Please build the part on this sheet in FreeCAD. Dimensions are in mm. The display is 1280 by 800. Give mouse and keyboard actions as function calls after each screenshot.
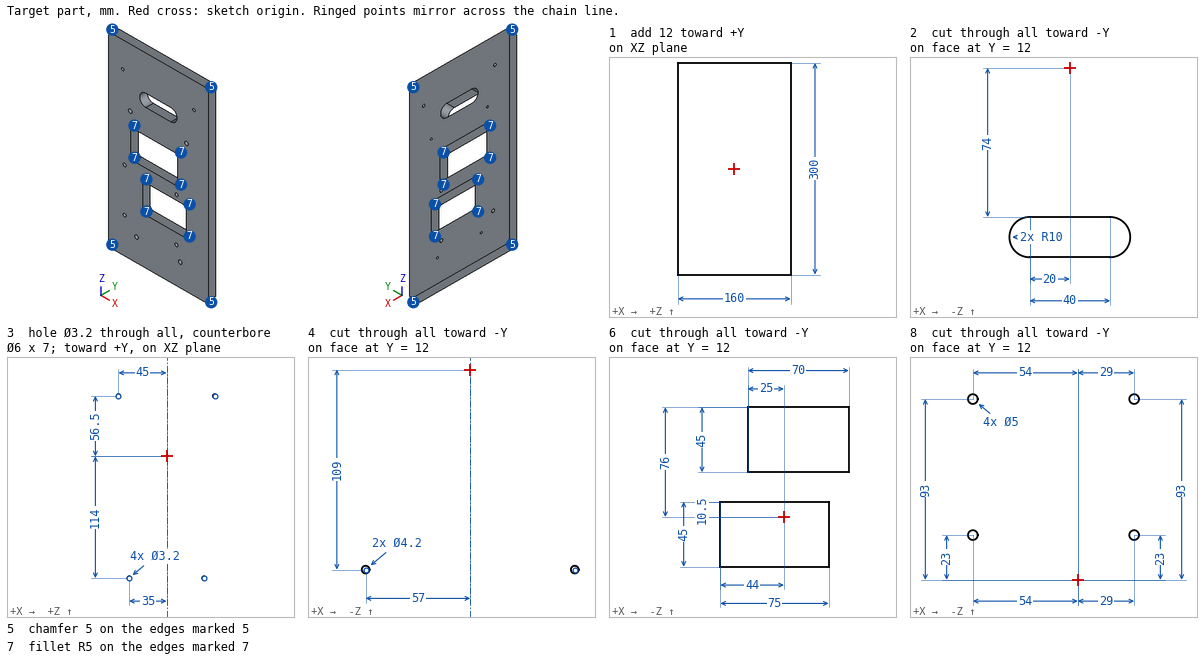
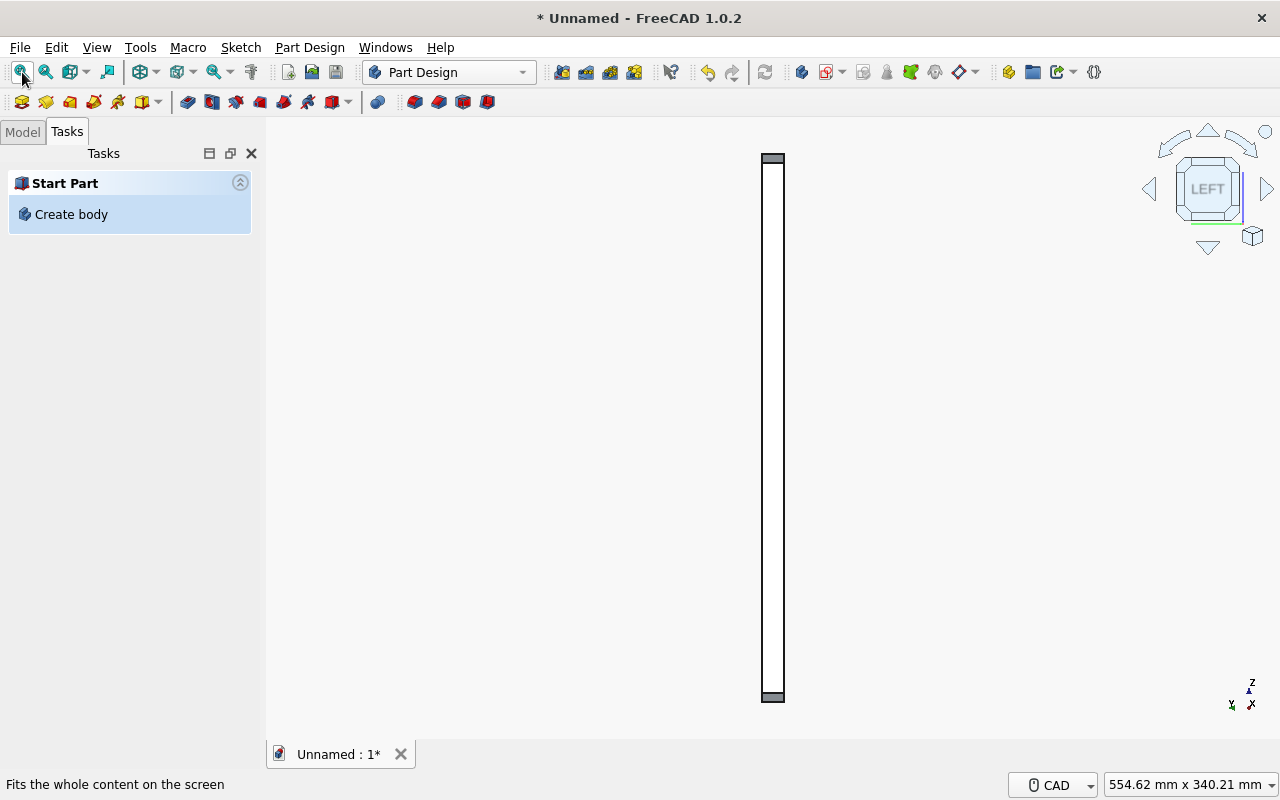
key(0)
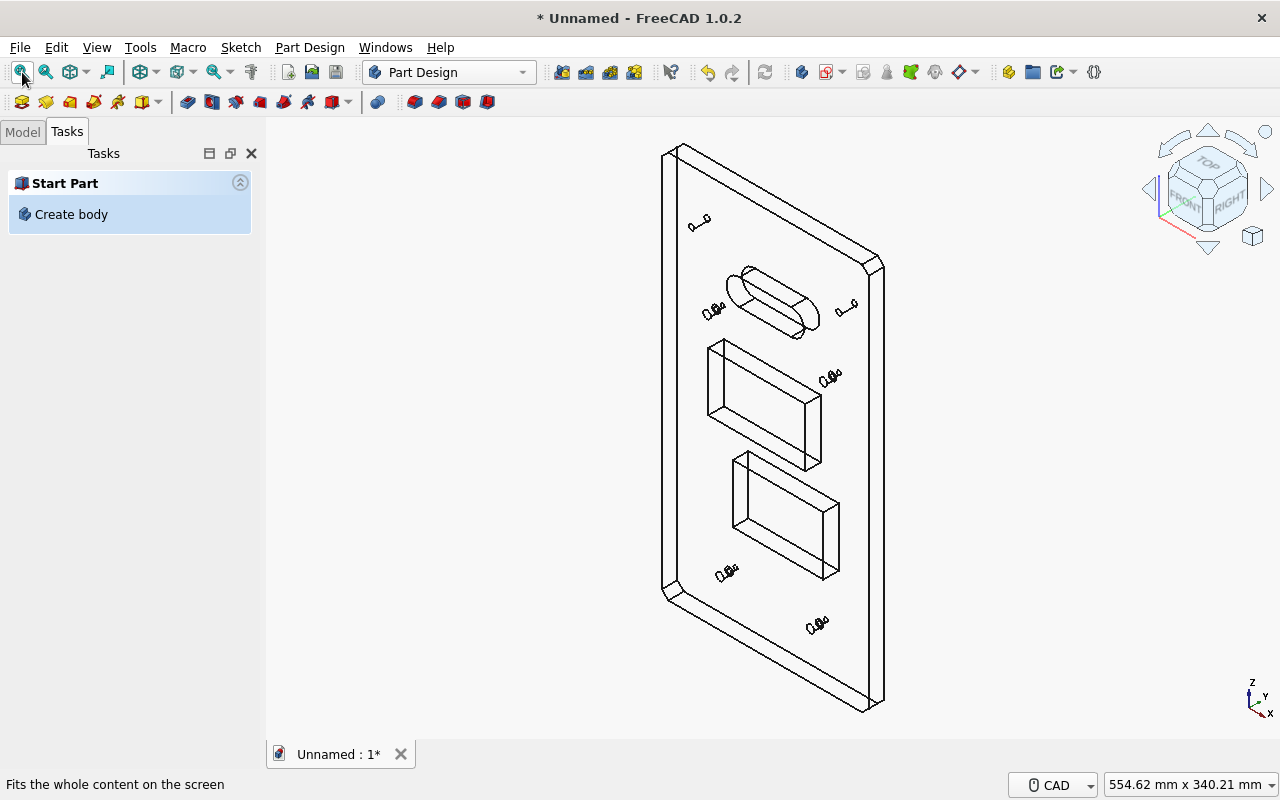
click(813, 466)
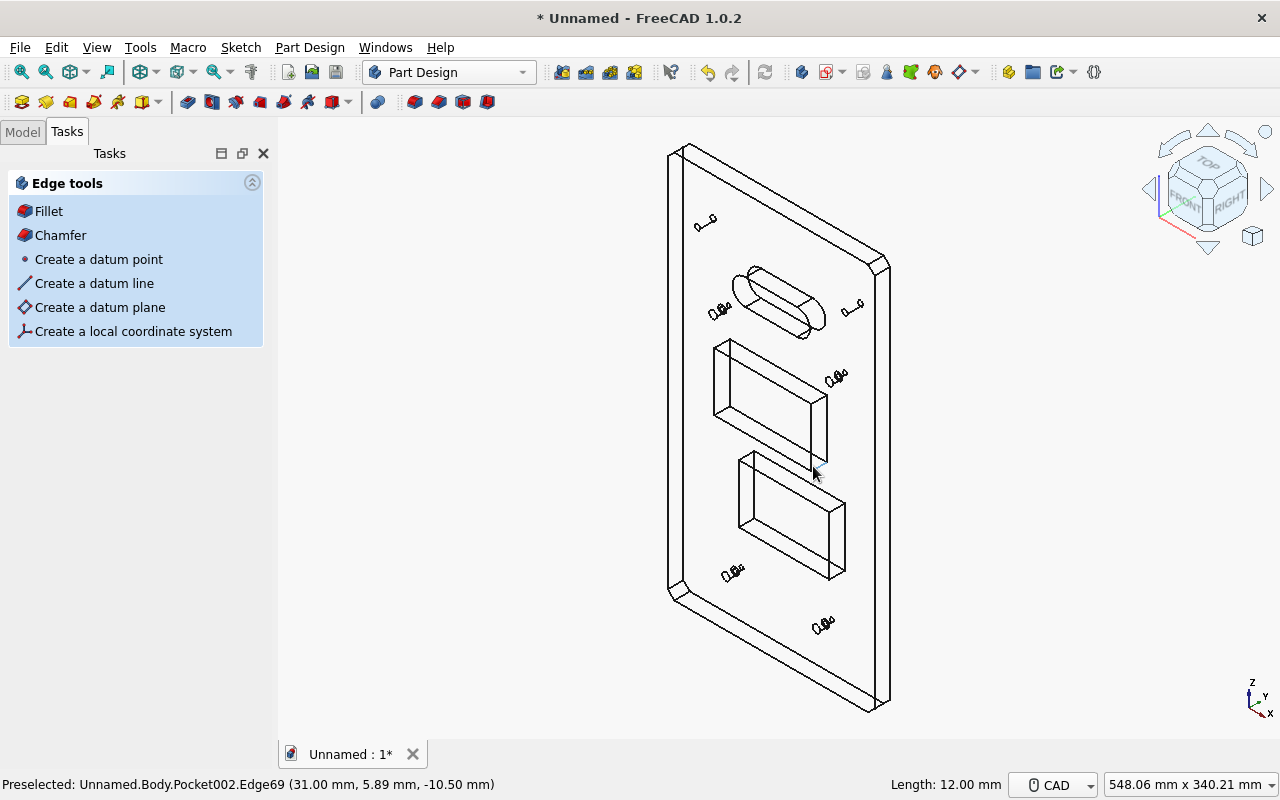
click(819, 399, ctrl)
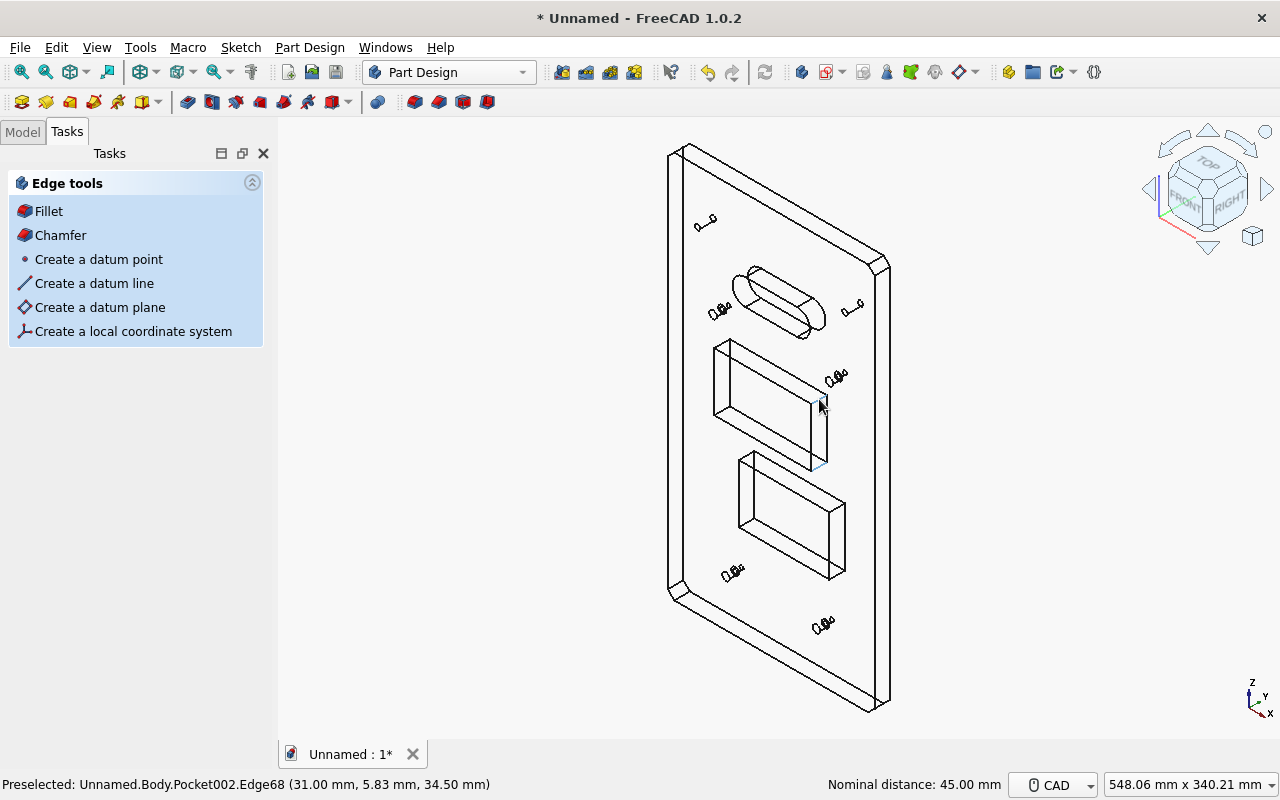
click(722, 343, ctrl)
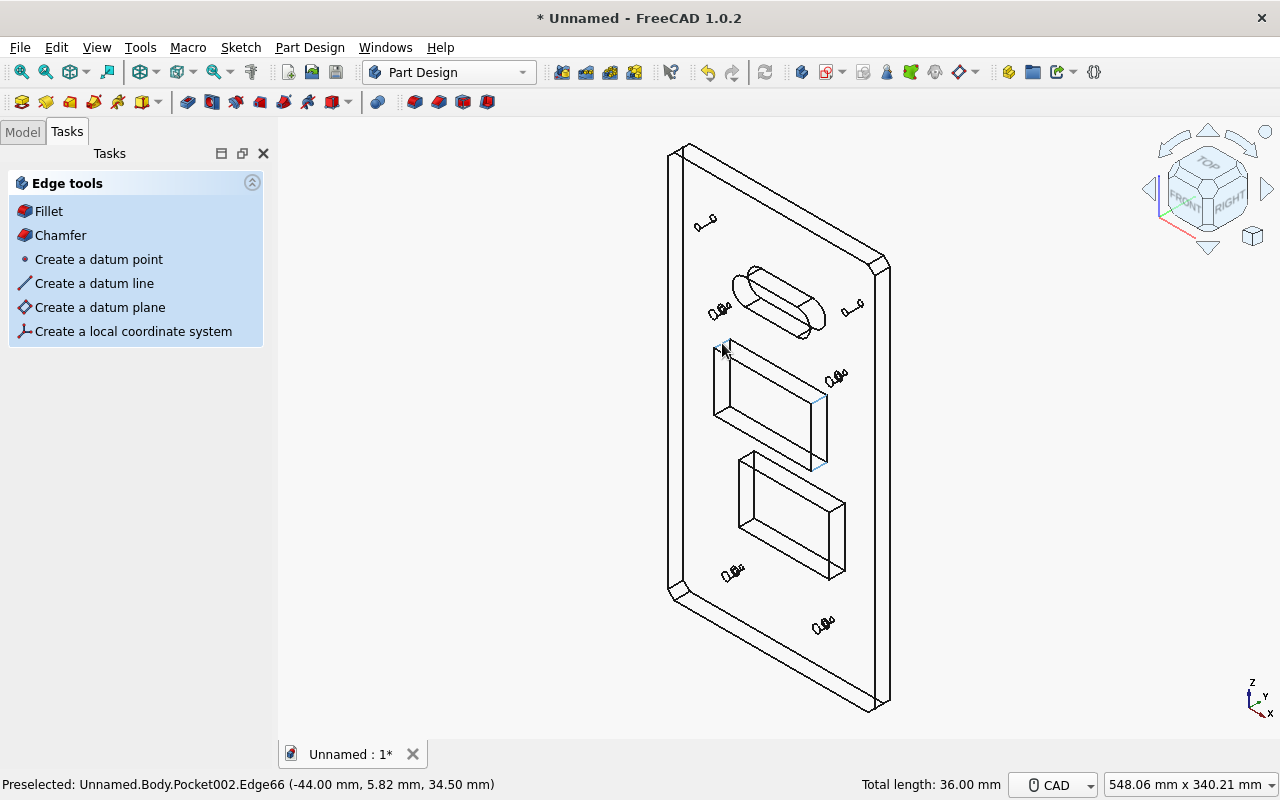
click(722, 410, ctrl)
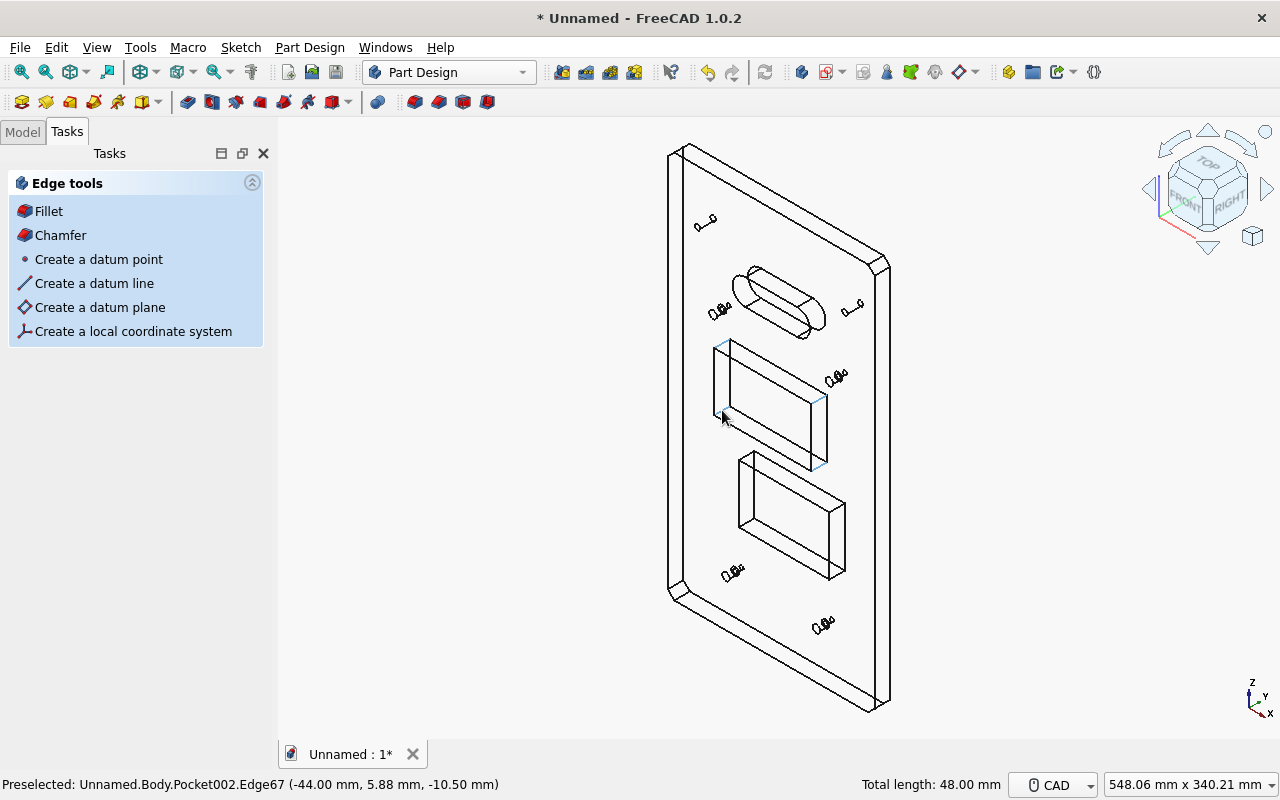
click(837, 574, ctrl)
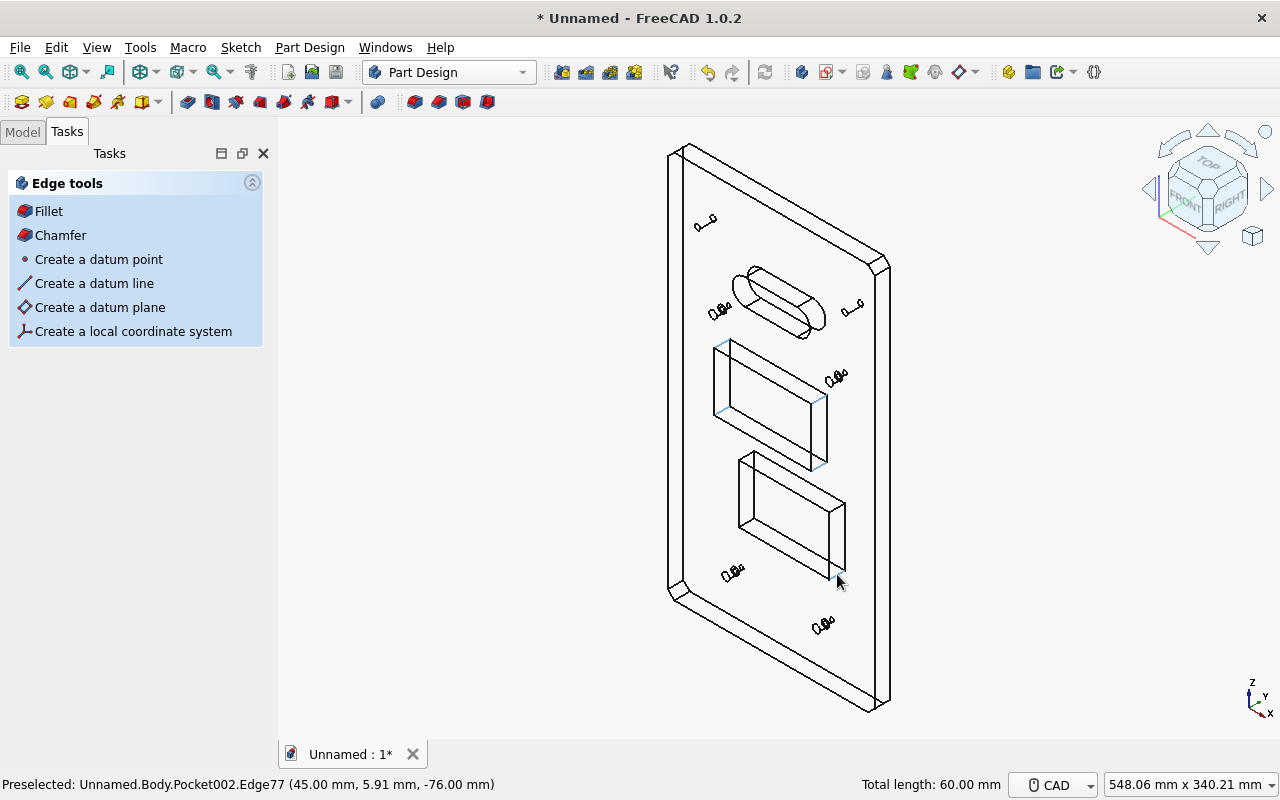
click(837, 507, ctrl)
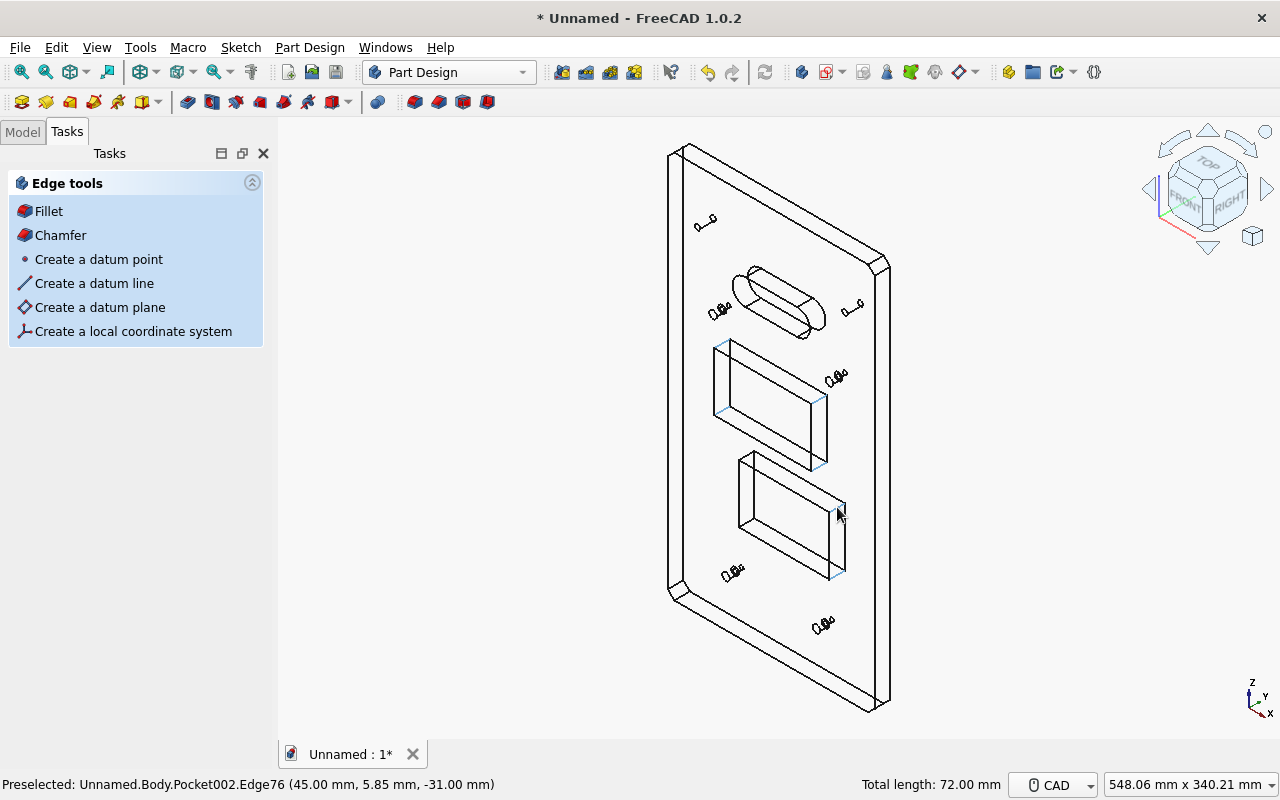
click(747, 455, ctrl)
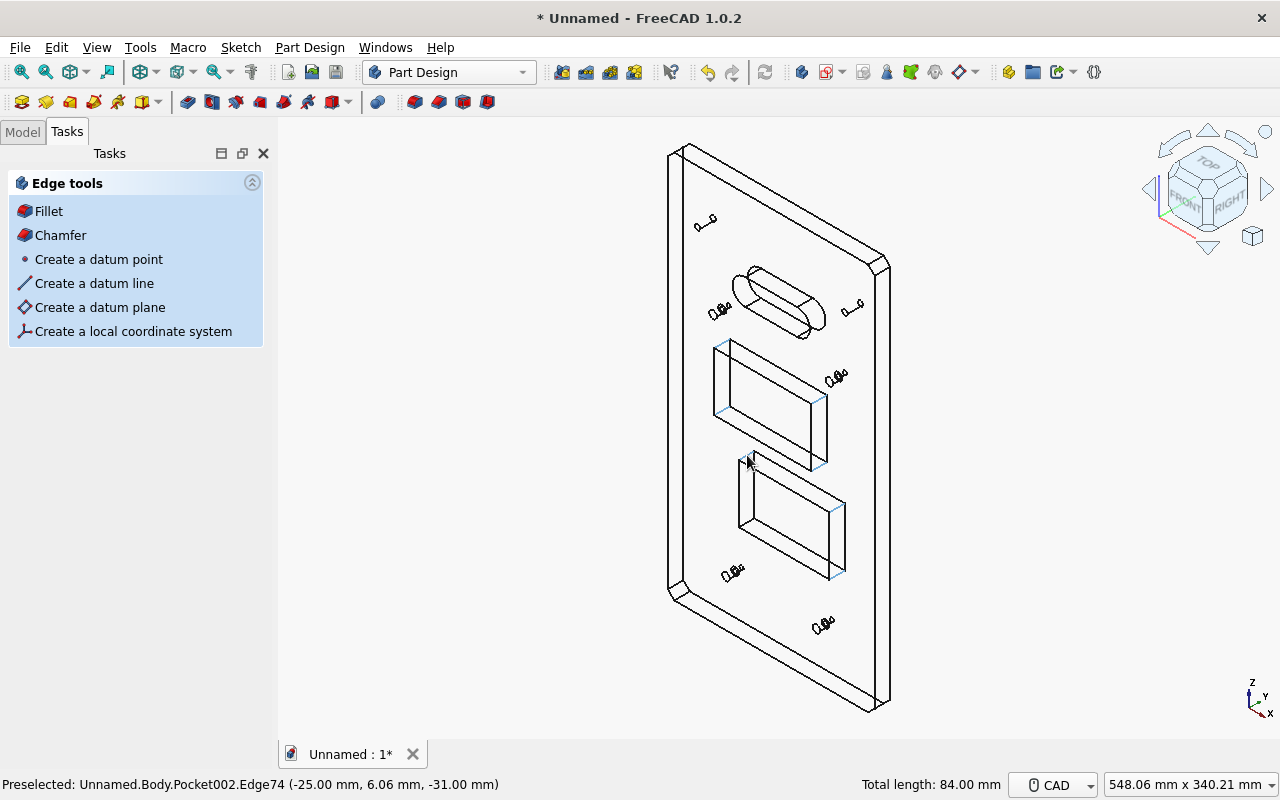
click(747, 522, ctrl)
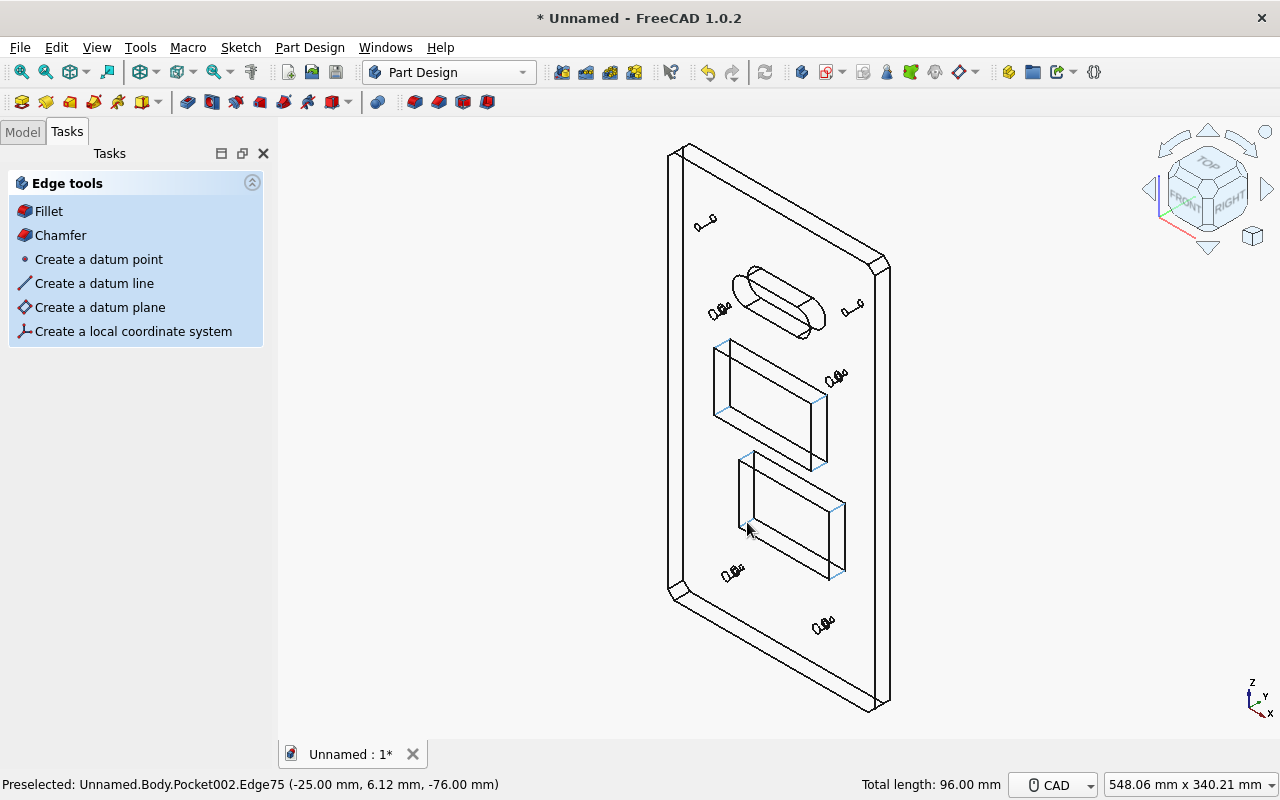
key(v)
key(1)